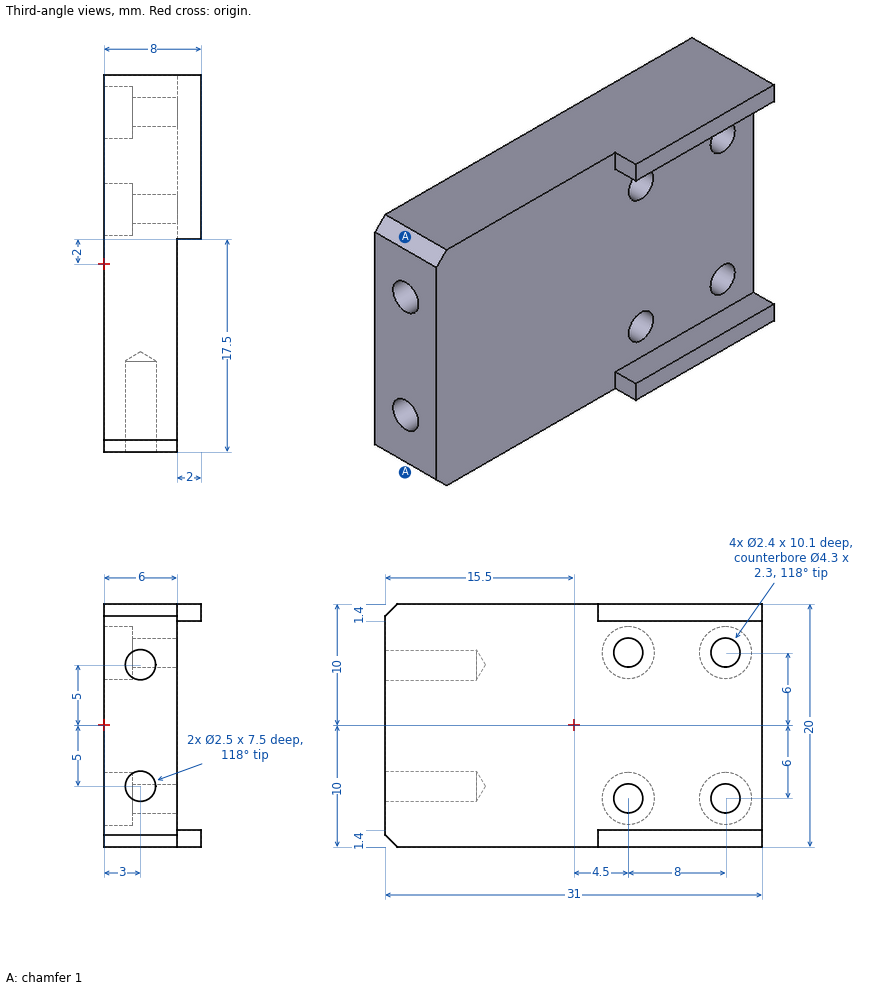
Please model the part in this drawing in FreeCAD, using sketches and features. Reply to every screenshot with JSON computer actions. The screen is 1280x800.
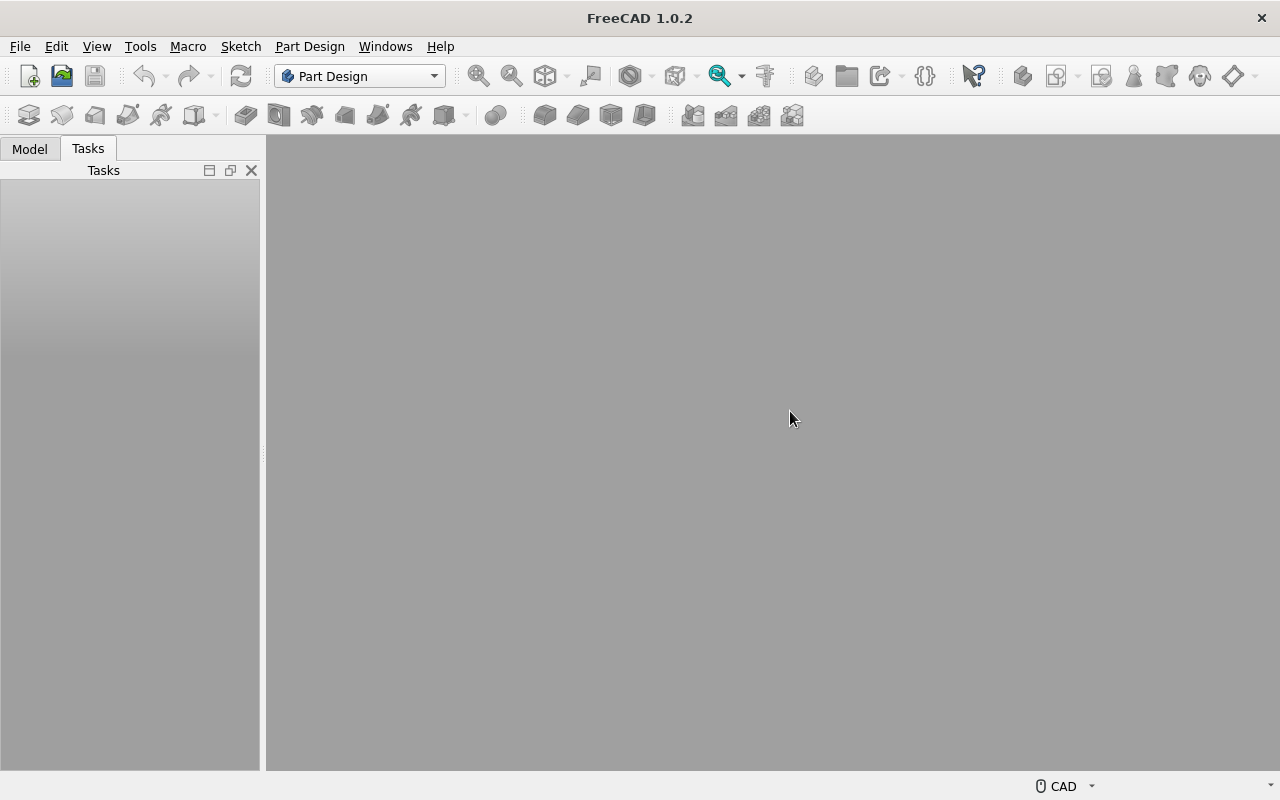
{"action": "left_click", "coordinate": [29, 76]}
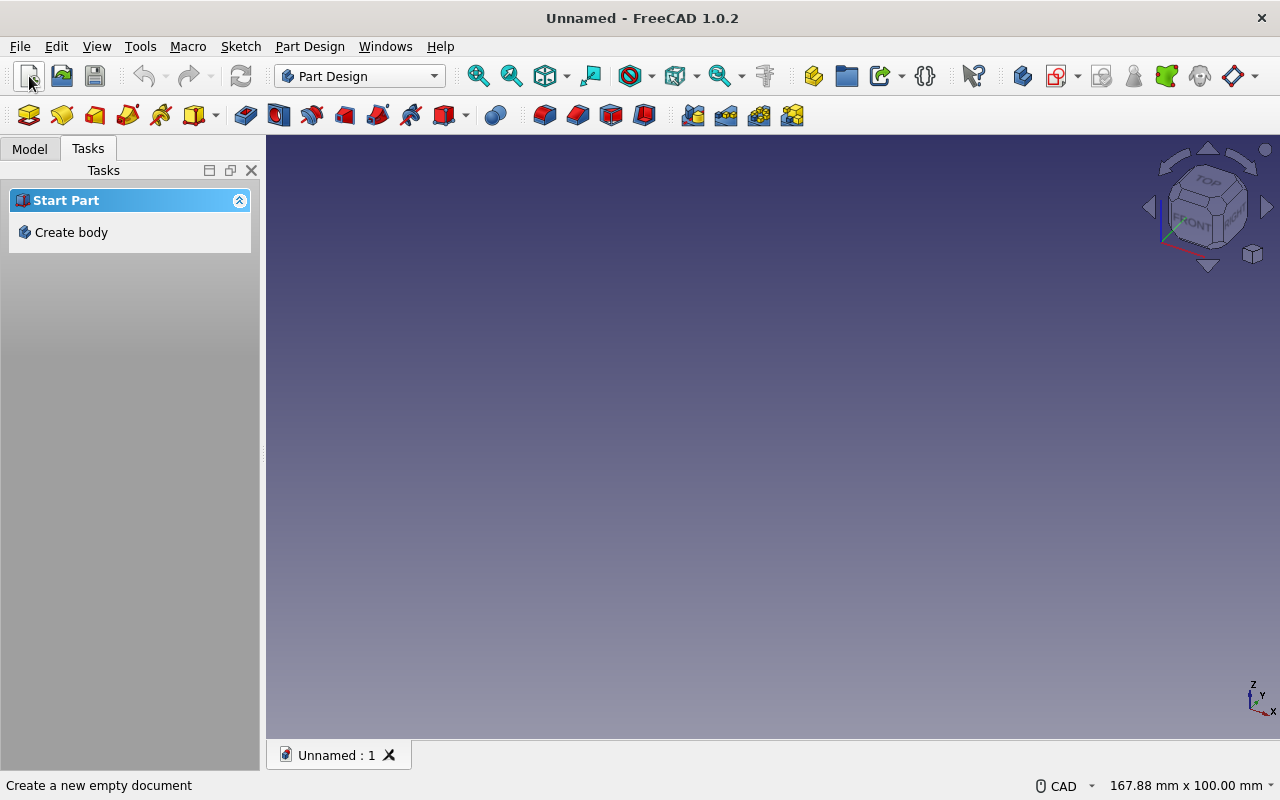
{"action": "left_click", "coordinate": [1056, 76]}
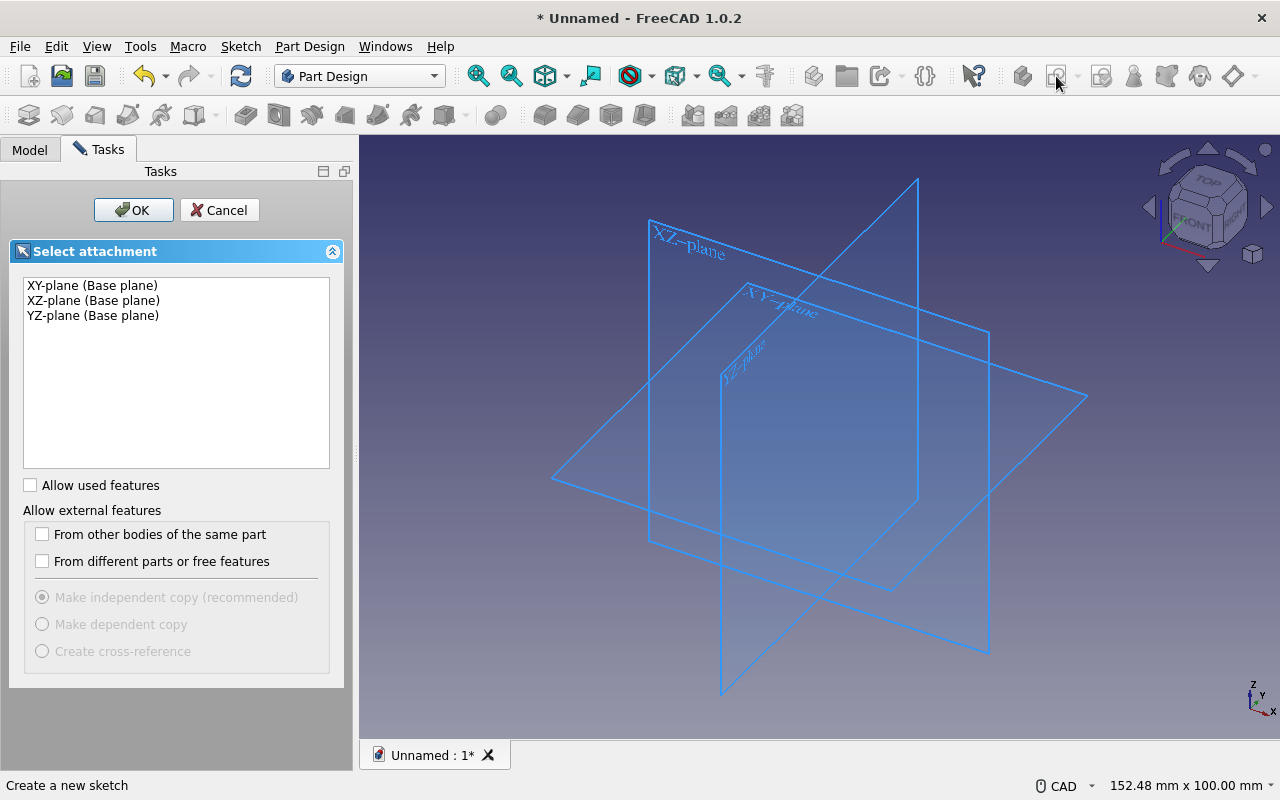
{"action": "left_click", "coordinate": [84, 316]}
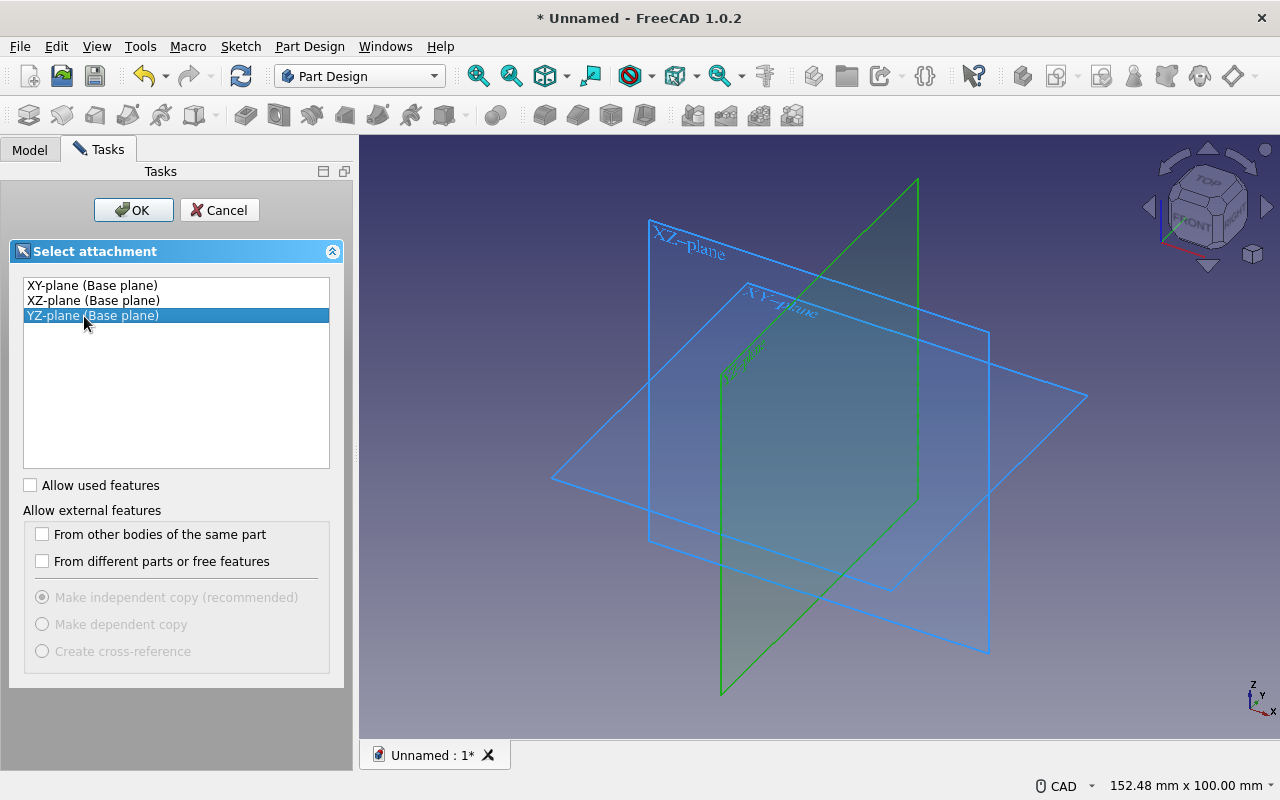
{"action": "left_click", "coordinate": [134, 210]}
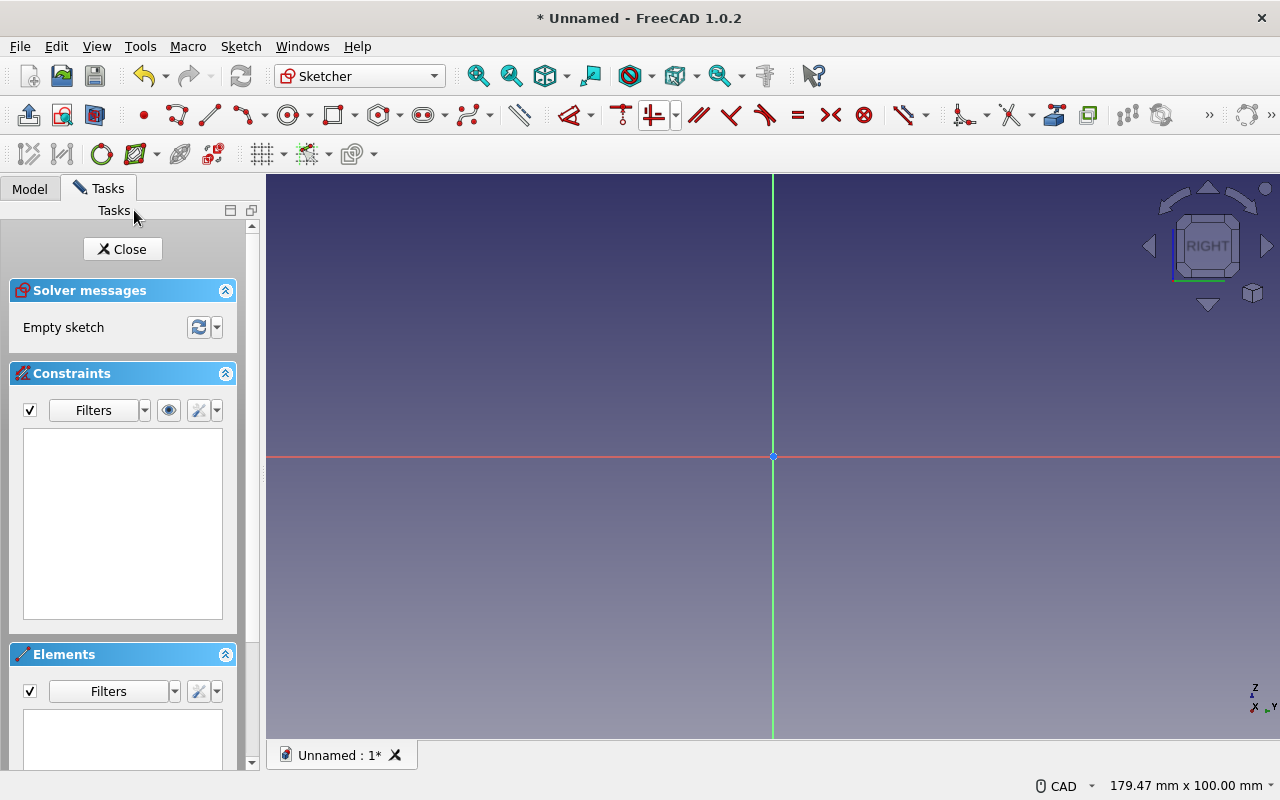
{"action": "scroll", "coordinate": [803, 456], "scroll_direction": "up", "scroll_amount": 6}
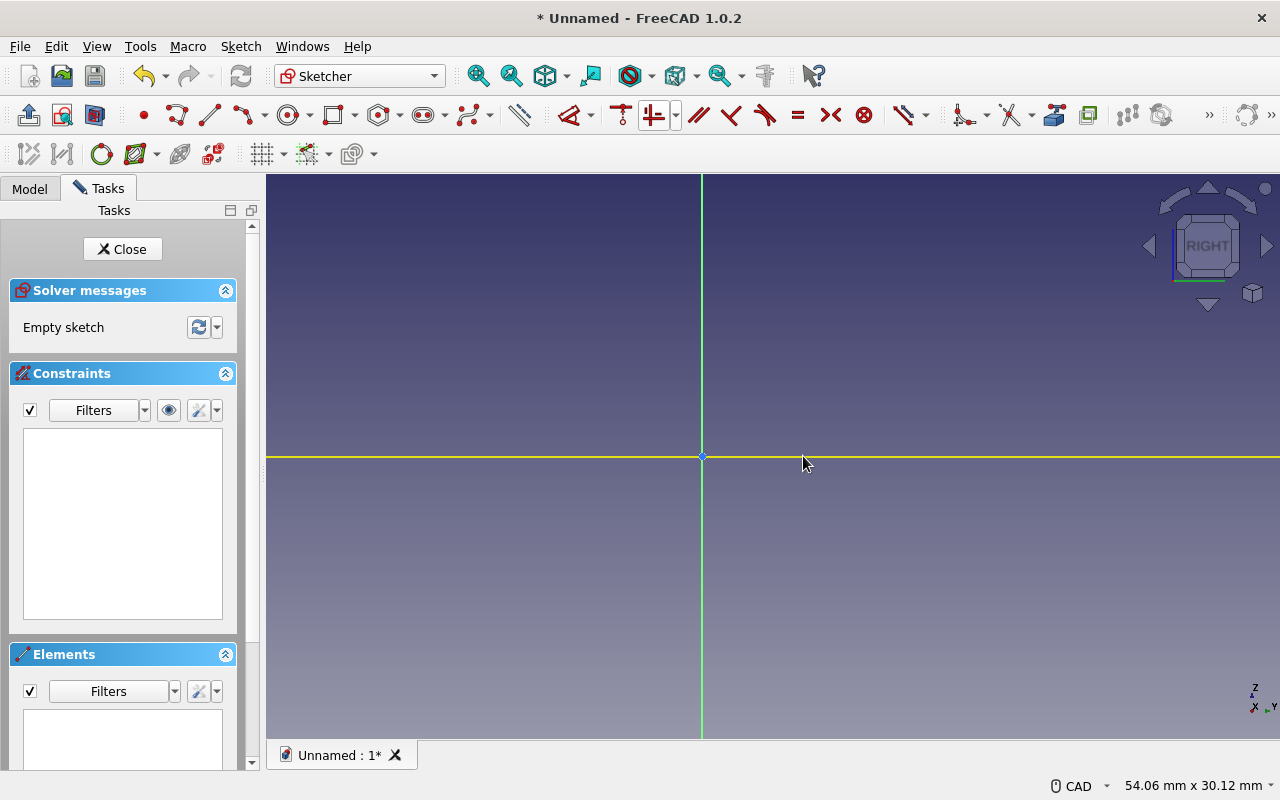
{"action": "left_click", "coordinate": [354, 116]}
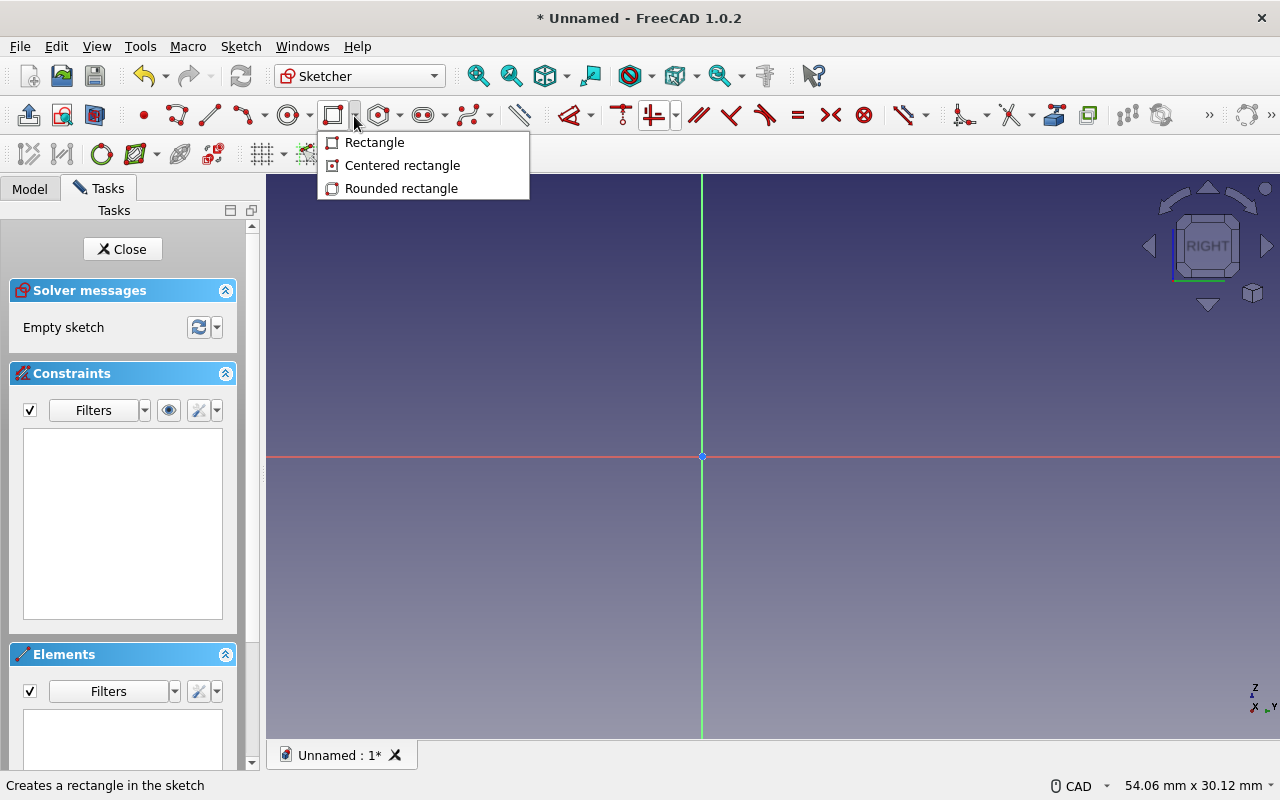
{"action": "left_click", "coordinate": [424, 166]}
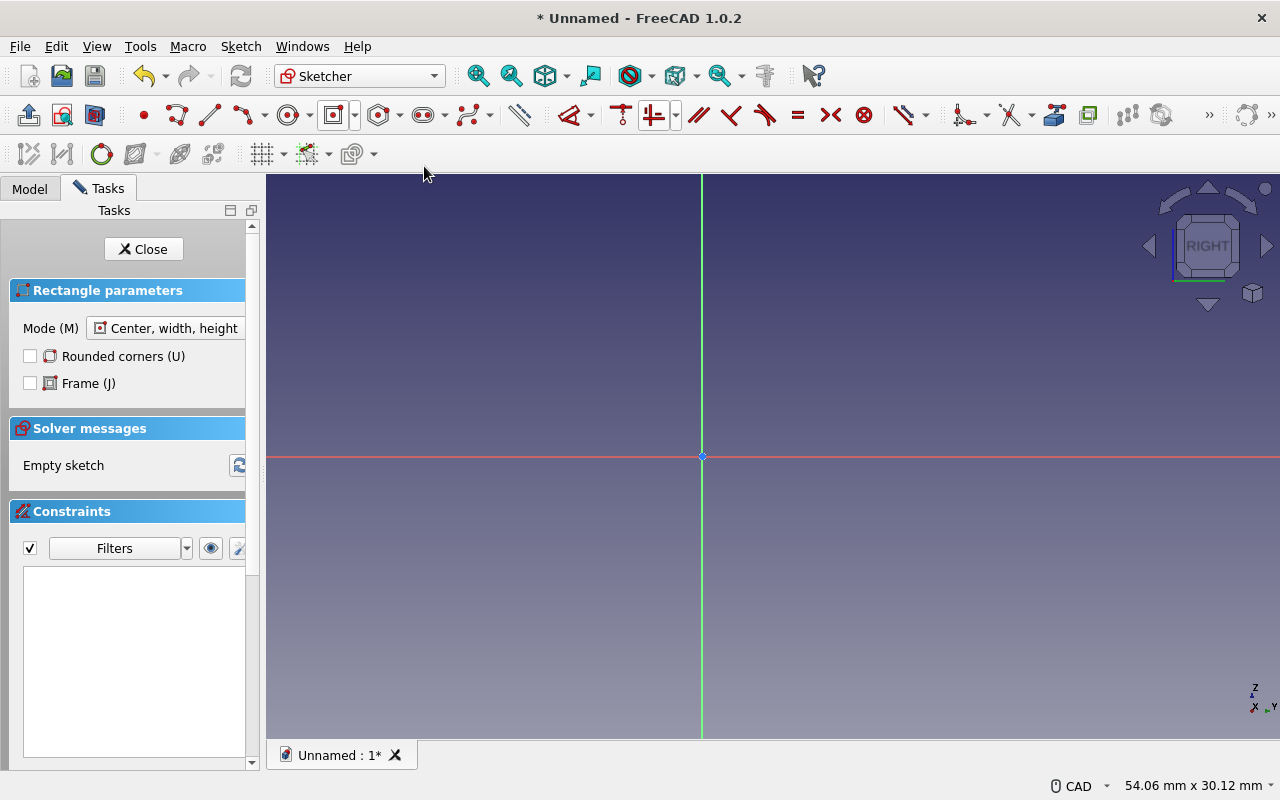
{"action": "left_click", "coordinate": [702, 456]}
{"action": "left_click", "coordinate": [993, 269]}
{"action": "key", "text": "Escape"}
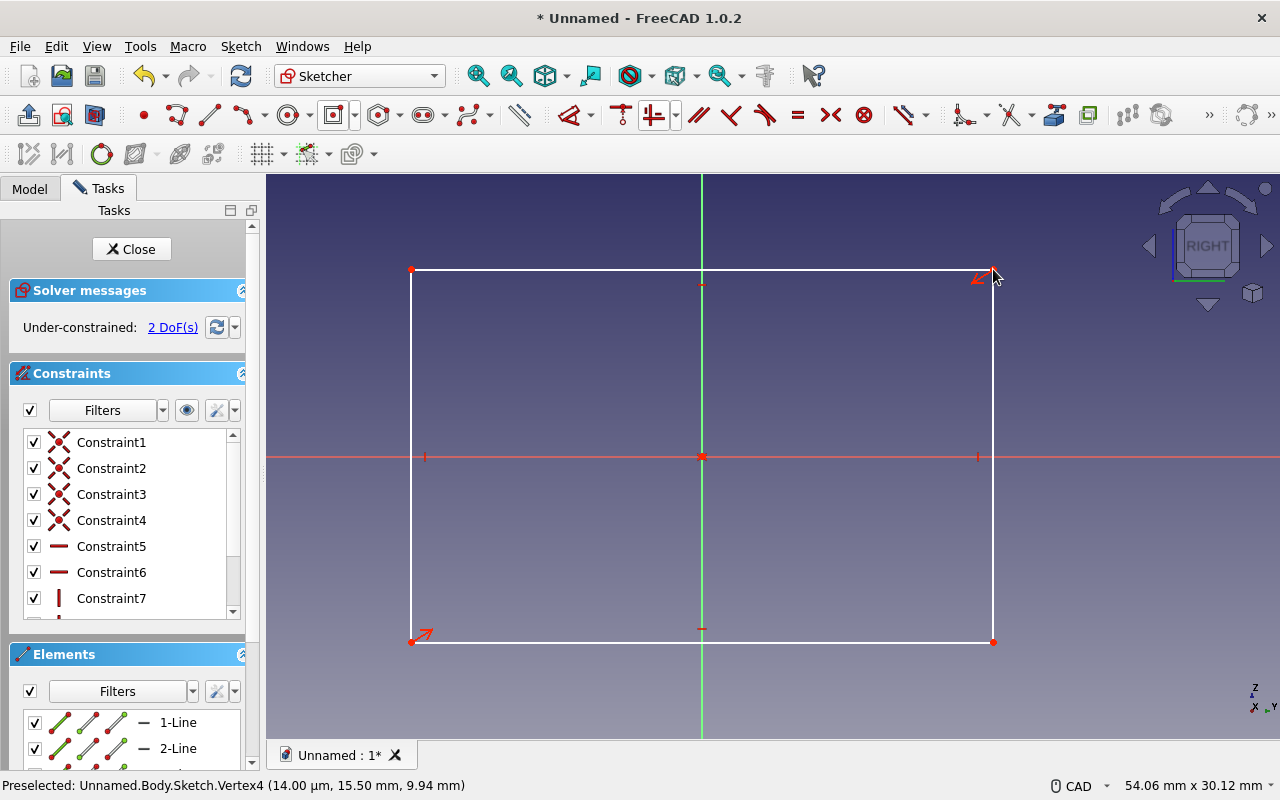
{"action": "left_click", "coordinate": [568, 116]}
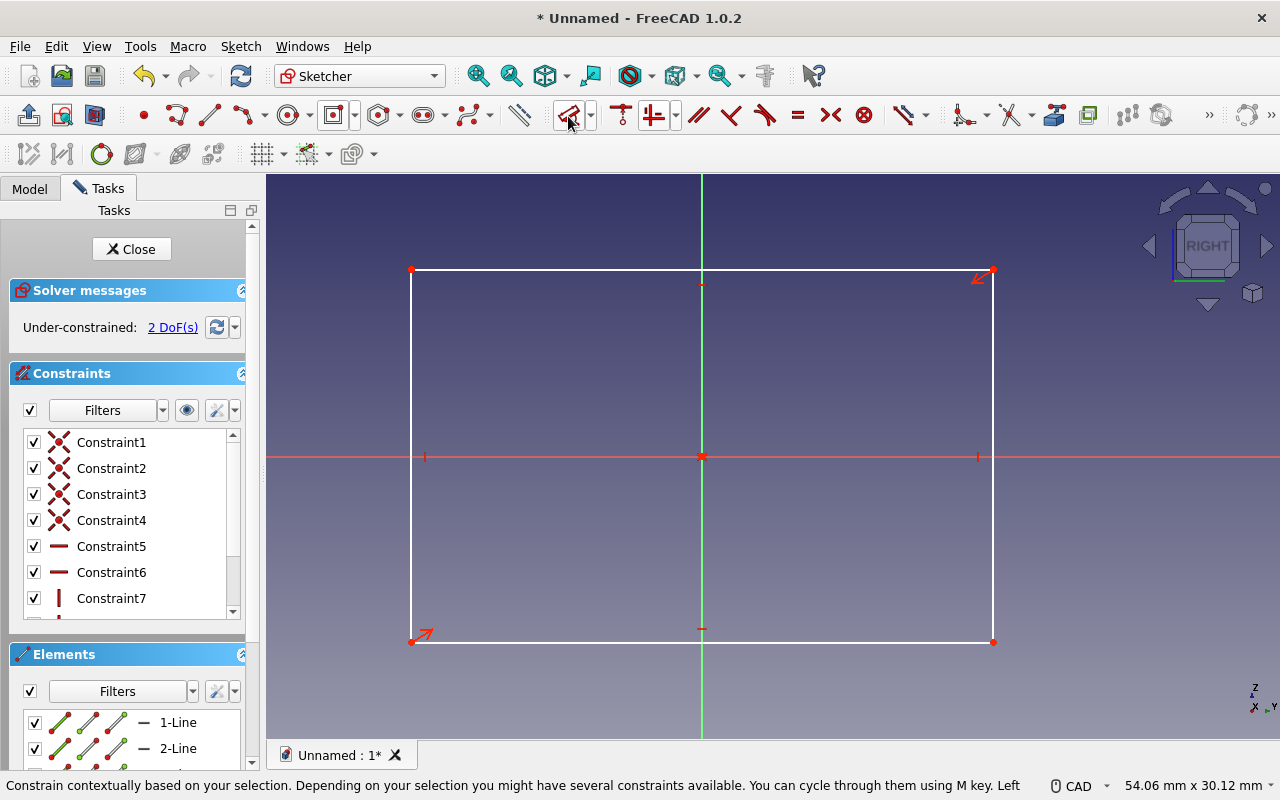
{"action": "left_click", "coordinate": [586, 643]}
{"action": "left_click", "coordinate": [568, 677]}